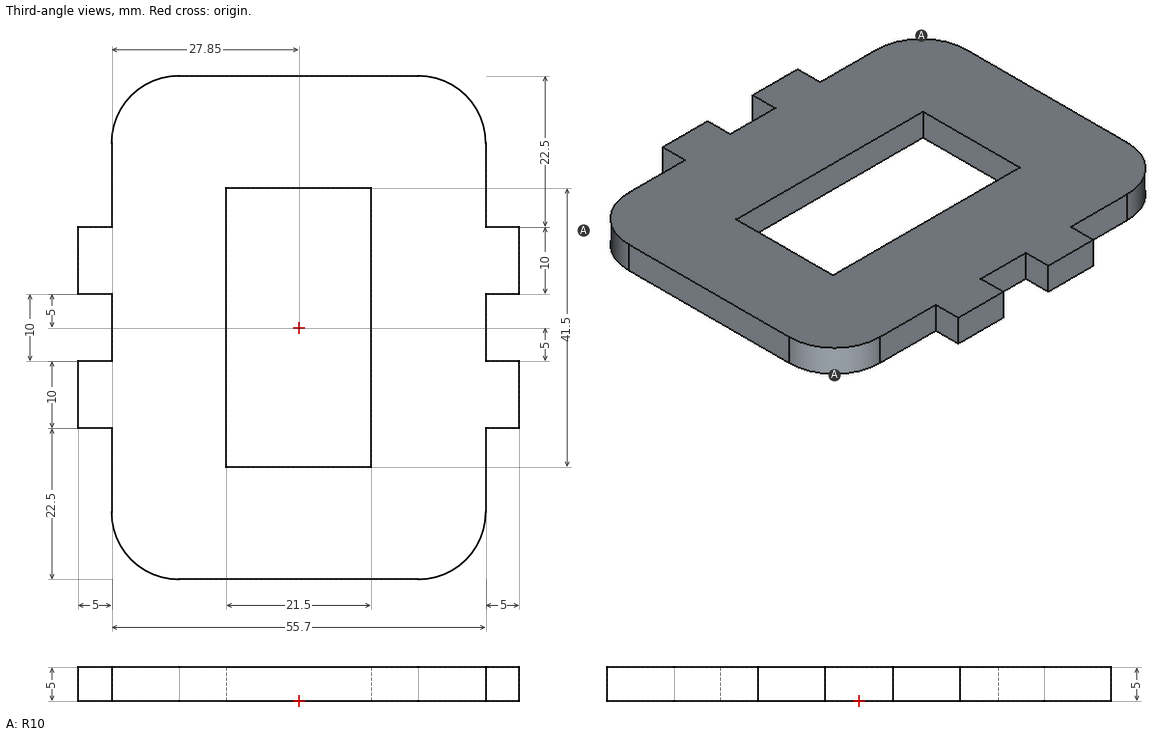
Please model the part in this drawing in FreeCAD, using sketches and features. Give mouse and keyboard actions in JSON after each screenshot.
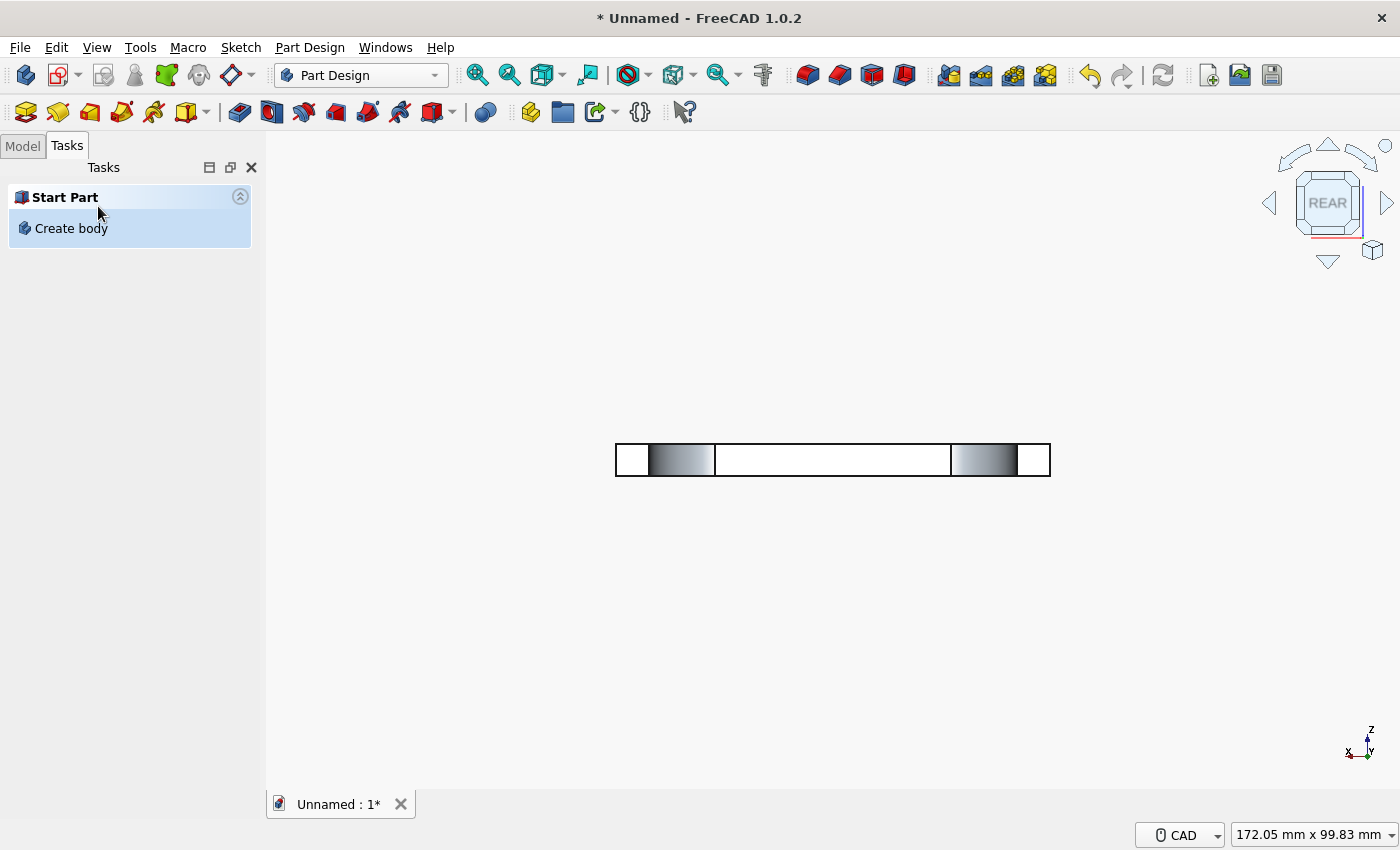
{"action": "key", "text": "0"}